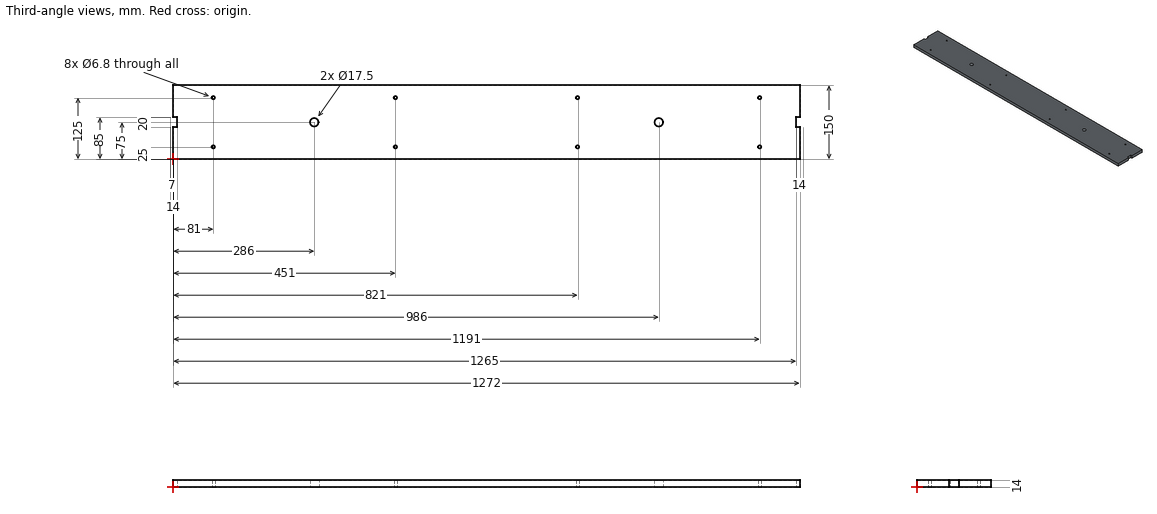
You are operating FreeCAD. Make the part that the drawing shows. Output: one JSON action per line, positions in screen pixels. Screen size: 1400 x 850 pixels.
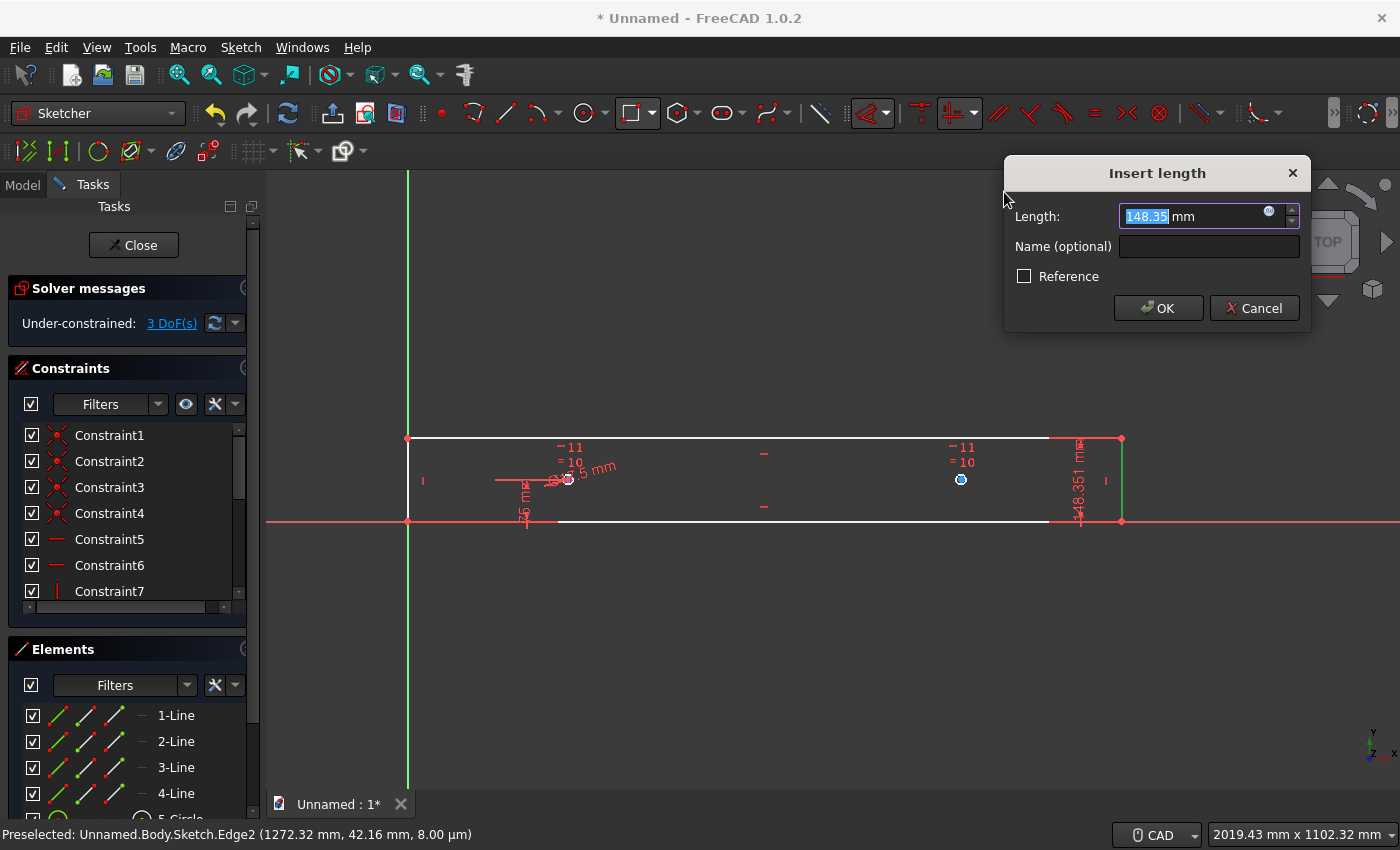
{"action": "type", "text": "150"}
{"action": "key", "text": "Return"}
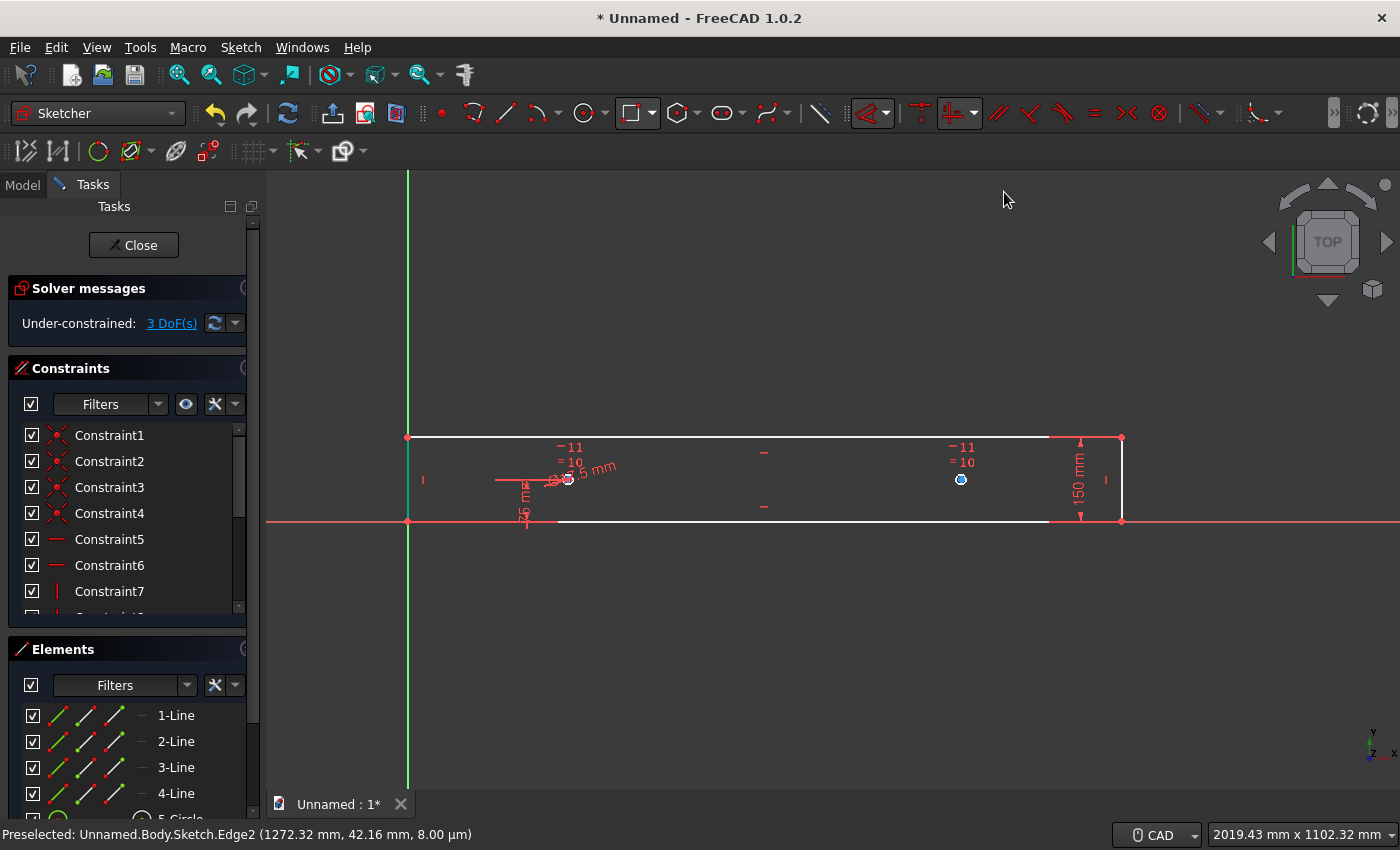
{"action": "left_click", "coordinate": [568, 480]}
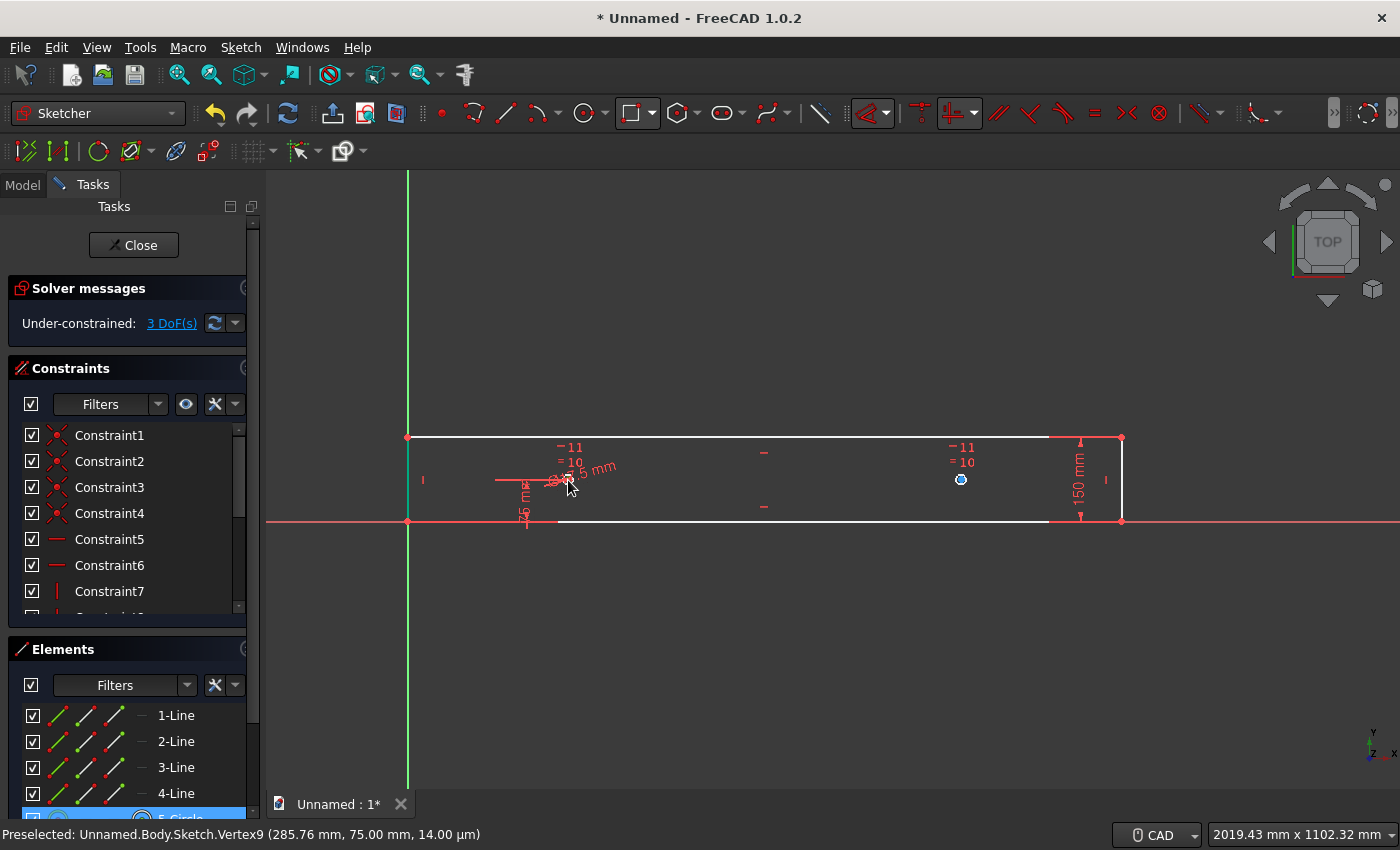
{"action": "key", "text": "l"}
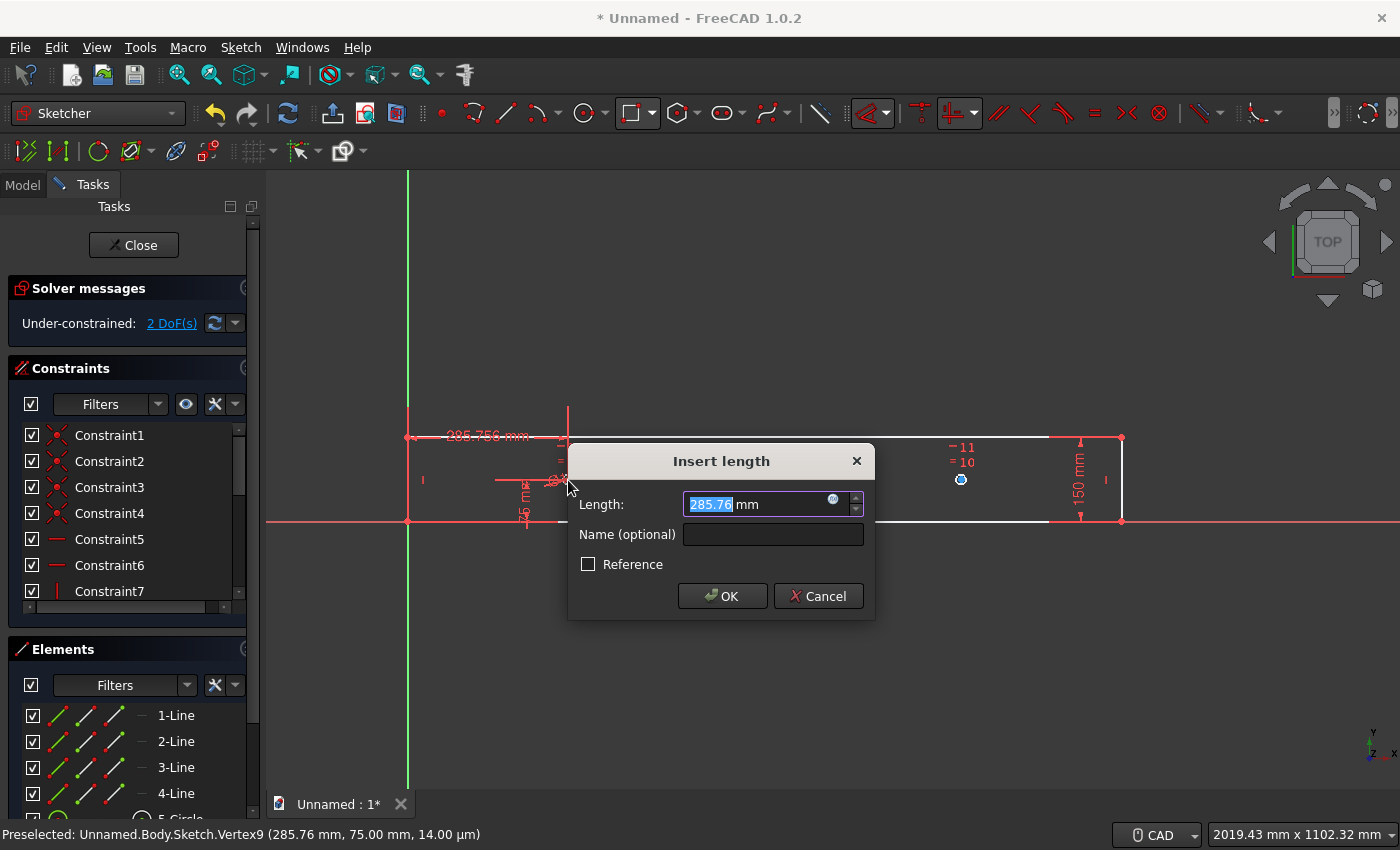
{"action": "type", "text": "286"}
{"action": "key", "text": "Return"}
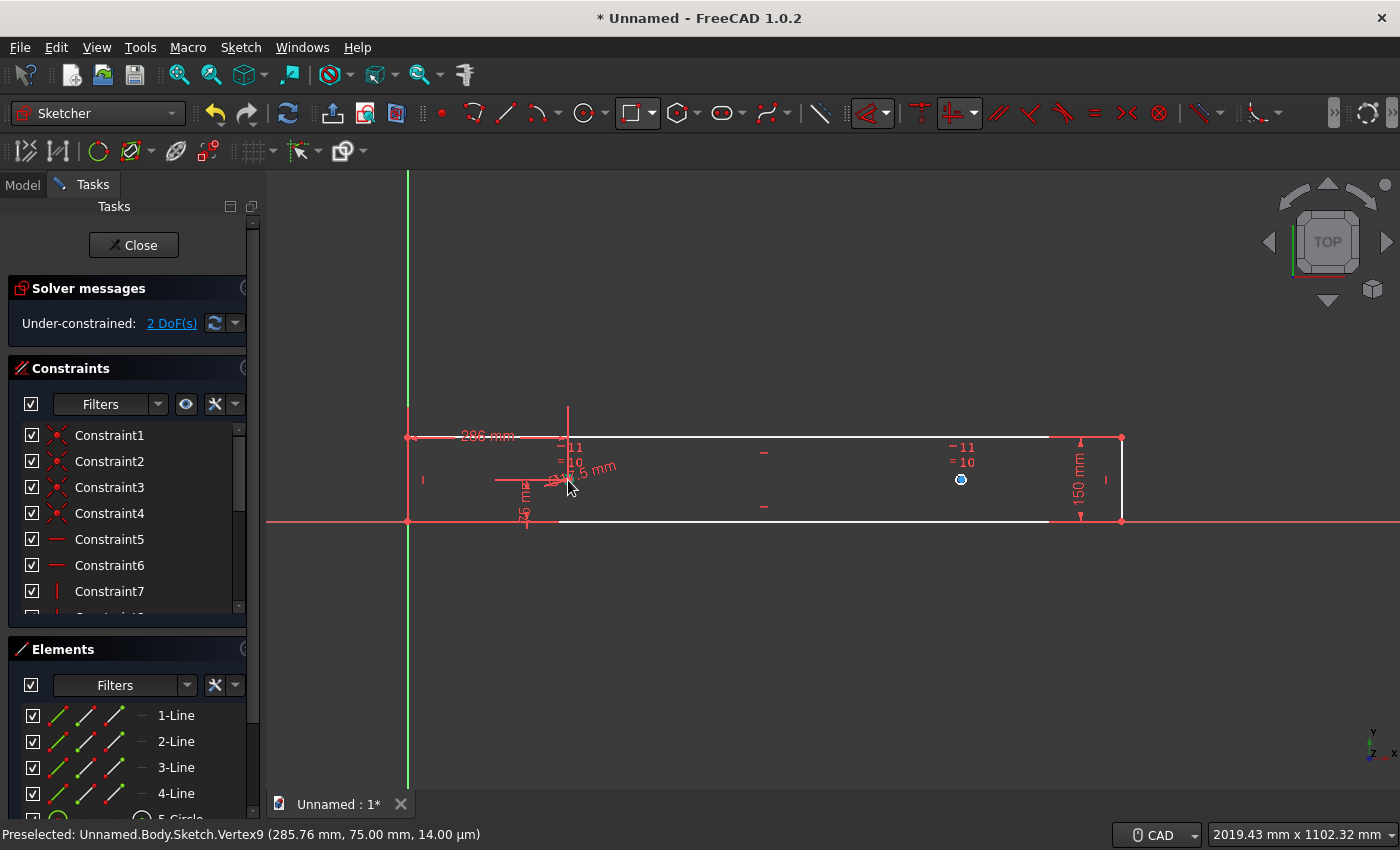
{"action": "left_click", "coordinate": [961, 480]}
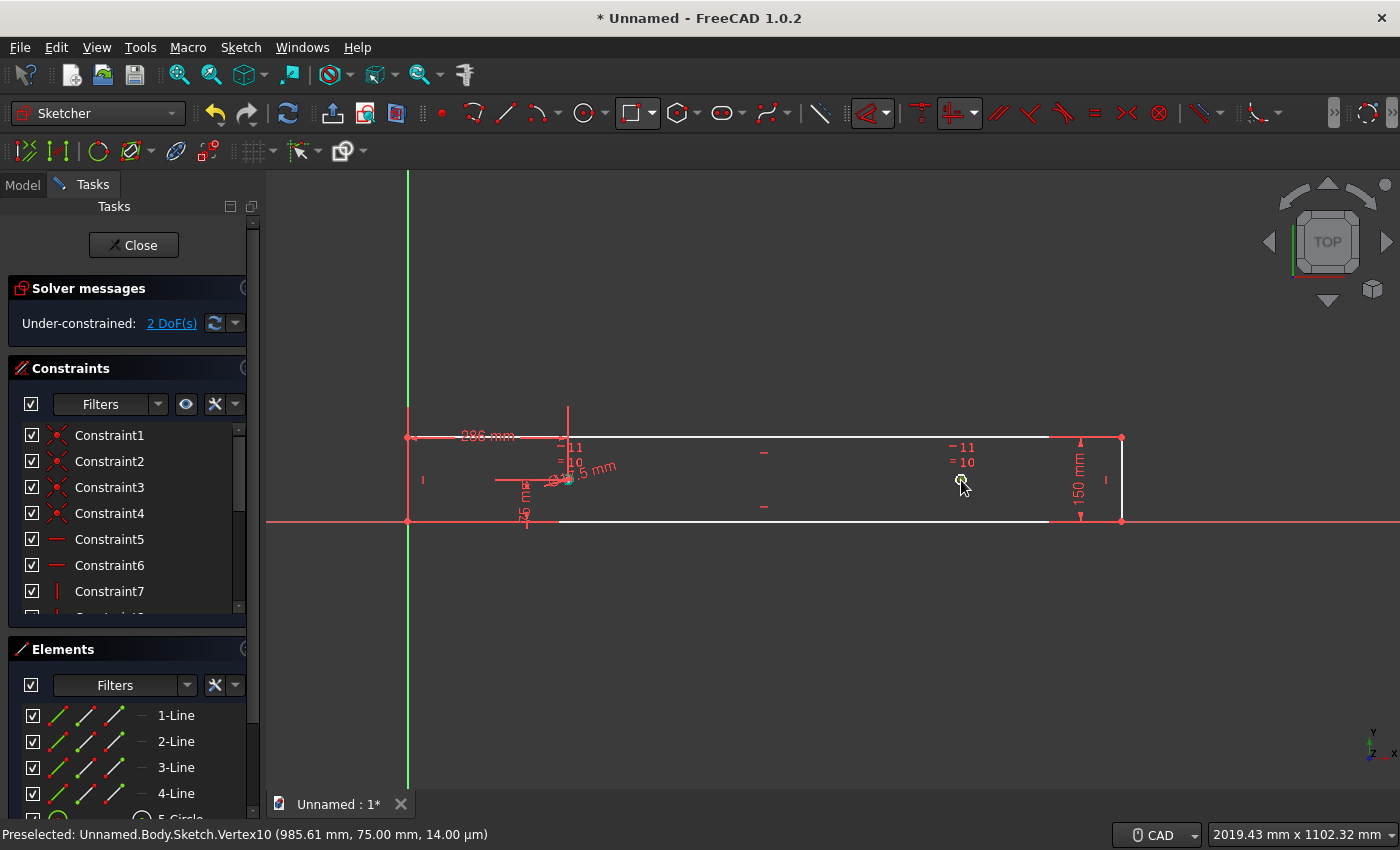
{"action": "key", "text": "l"}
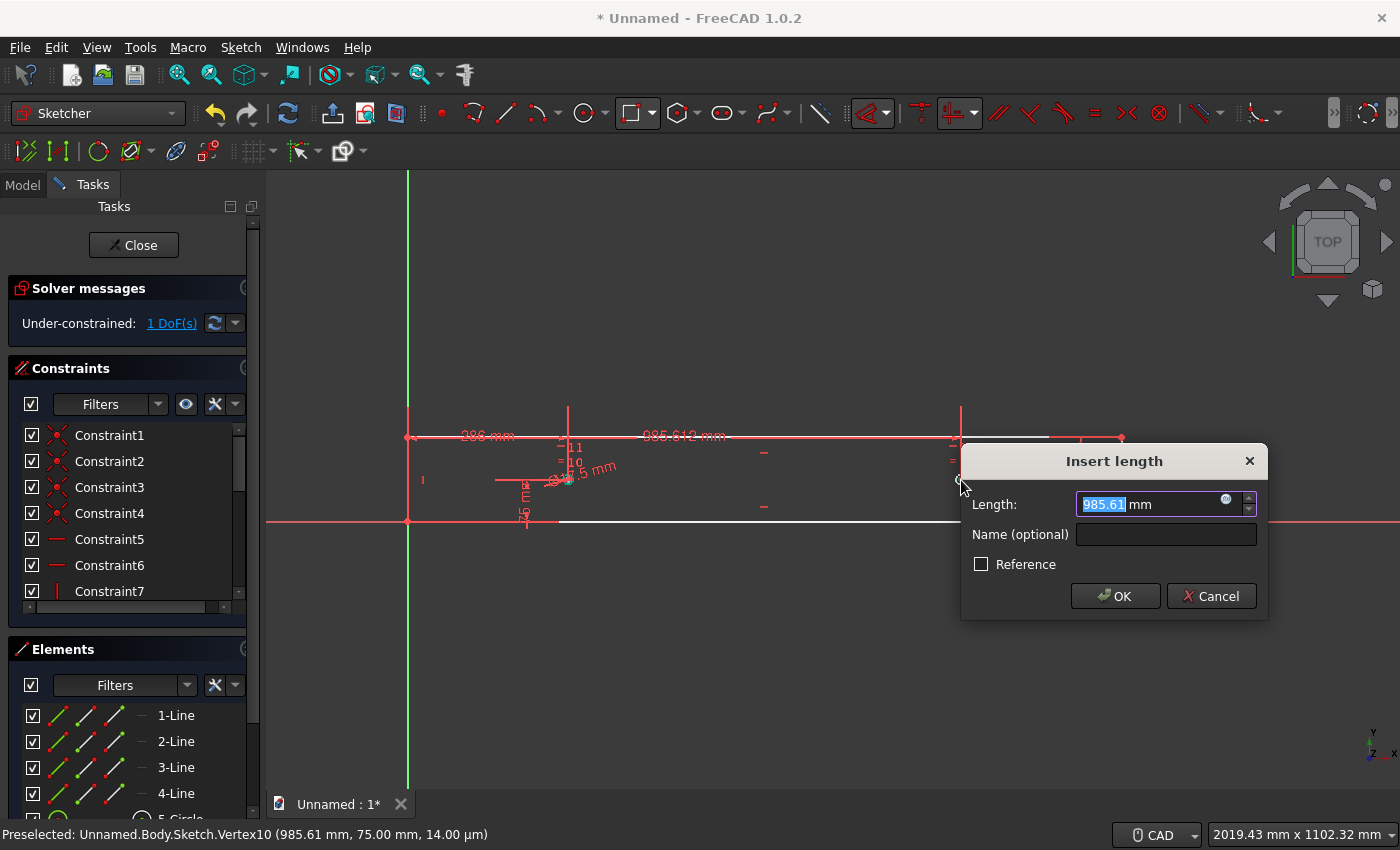
{"action": "type", "text": "986"}
{"action": "key", "text": "Return"}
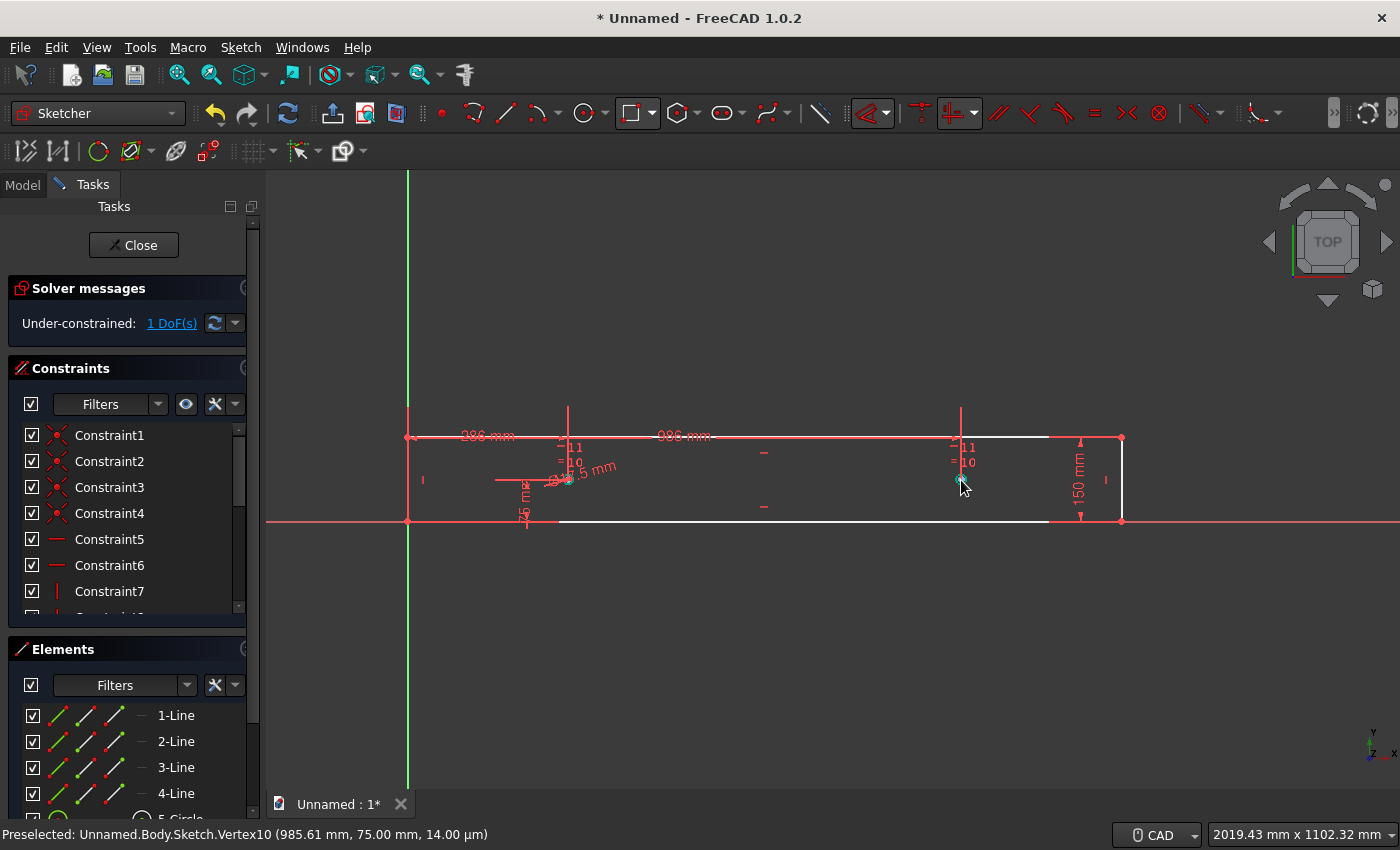
{"action": "left_click", "coordinate": [622, 522]}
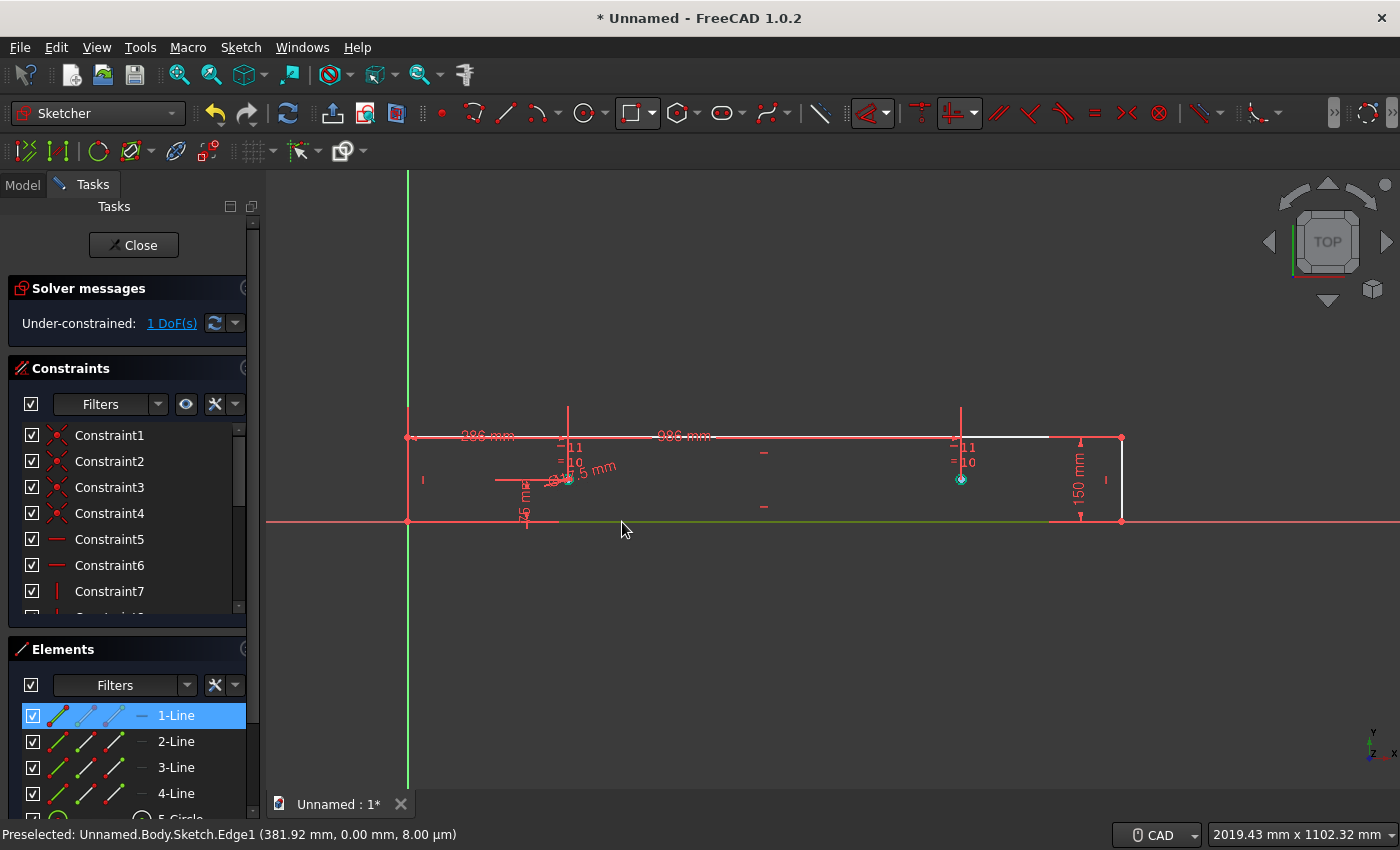
{"action": "left_click", "coordinate": [888, 114]}